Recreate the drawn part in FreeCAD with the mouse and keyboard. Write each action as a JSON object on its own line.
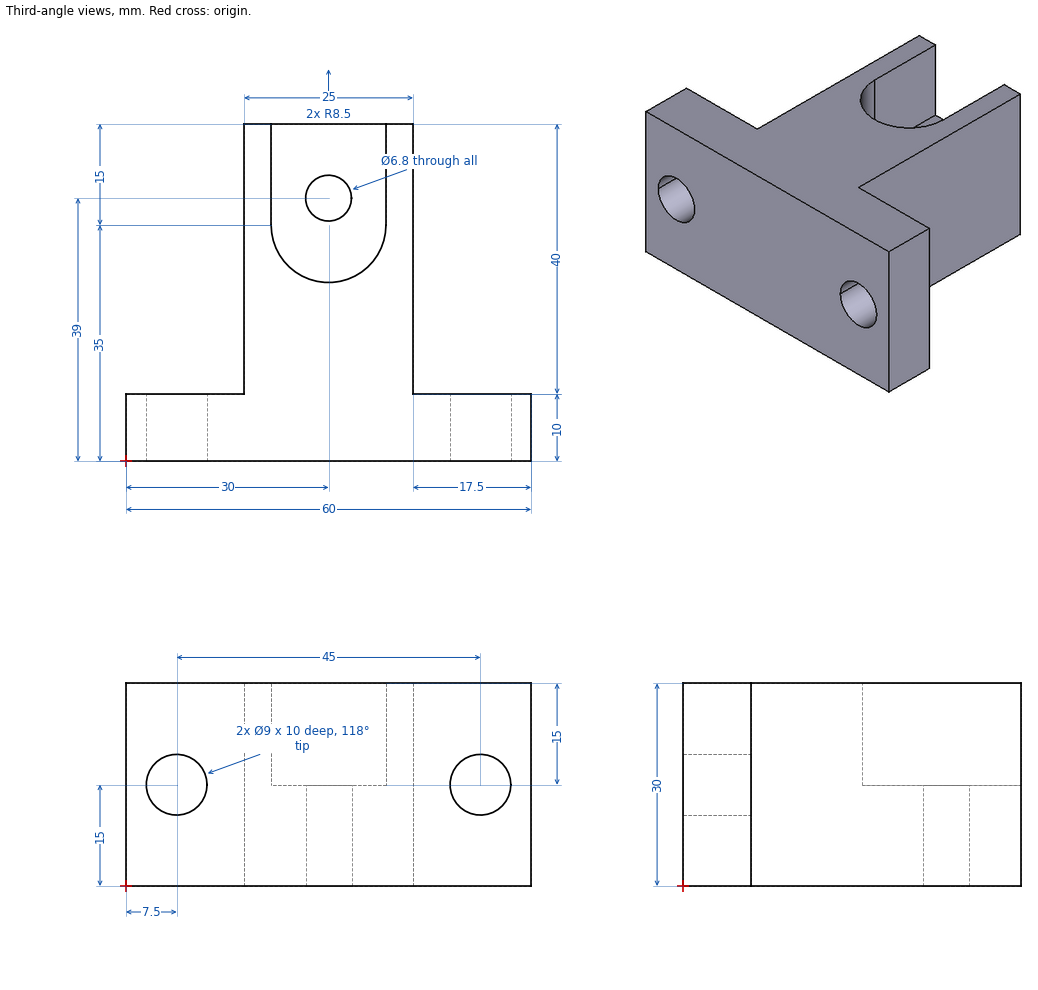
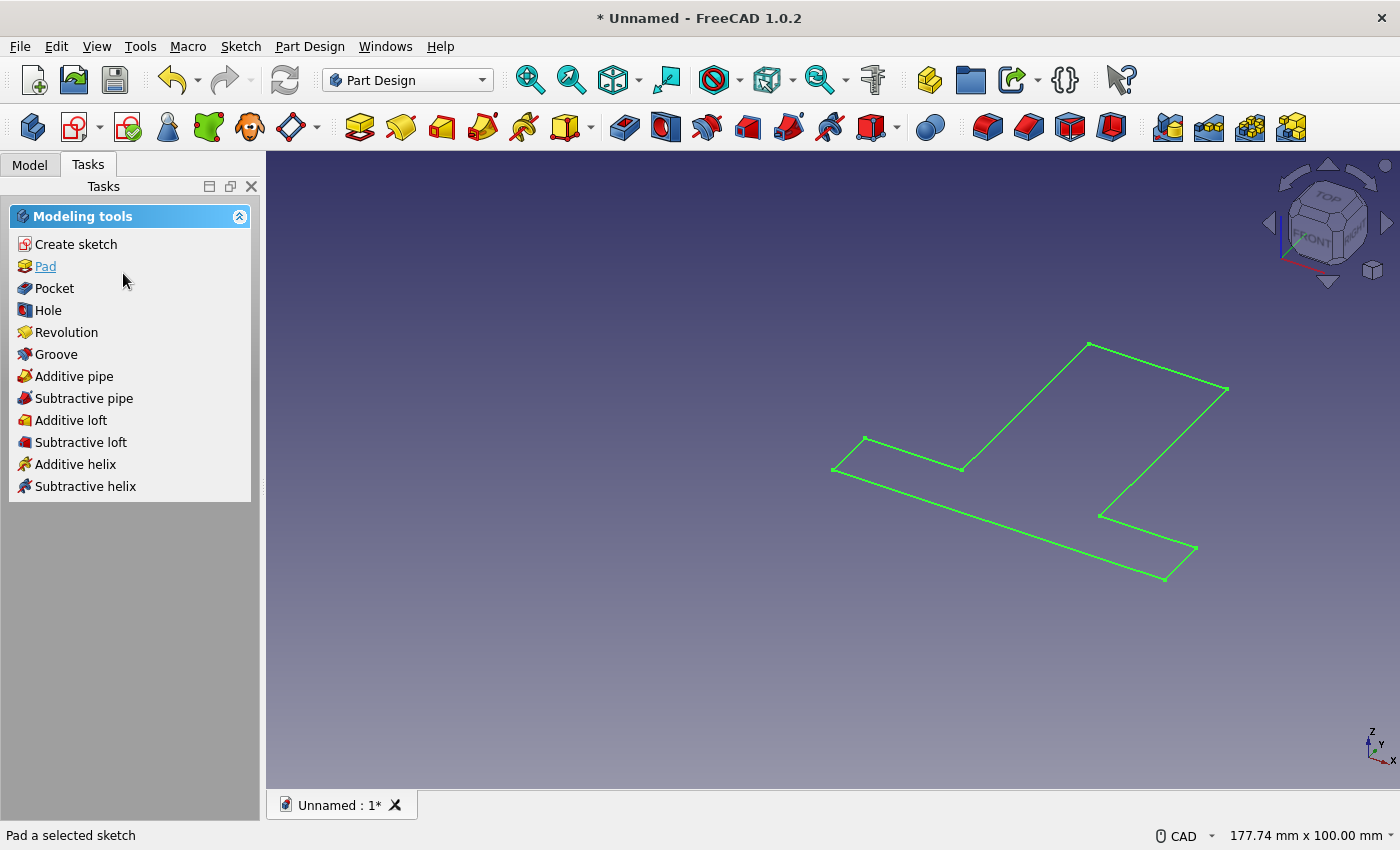
{"action": "left_click", "coordinate": [360, 128]}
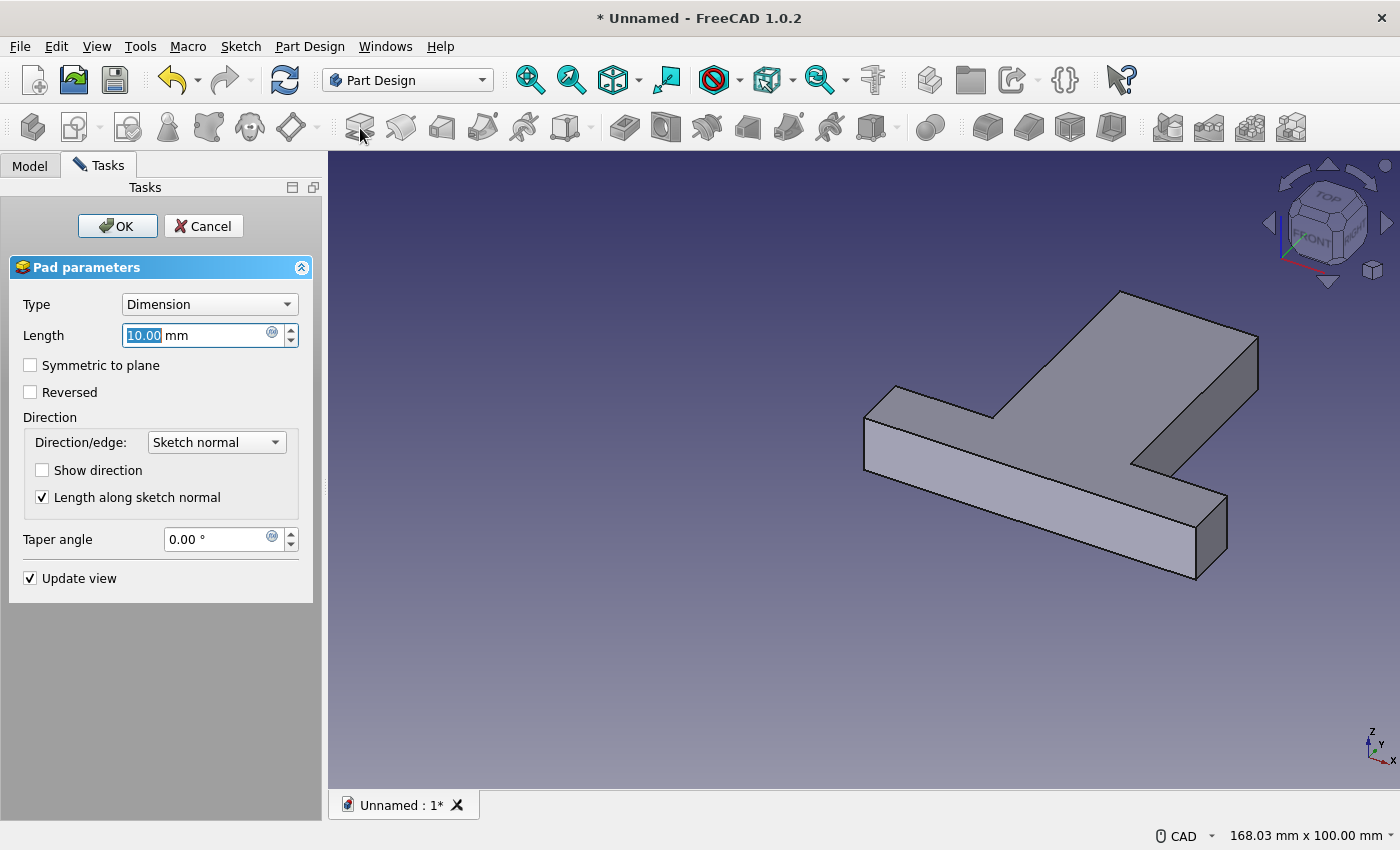
{"action": "type", "text": "30"}
{"action": "key", "text": "Tab"}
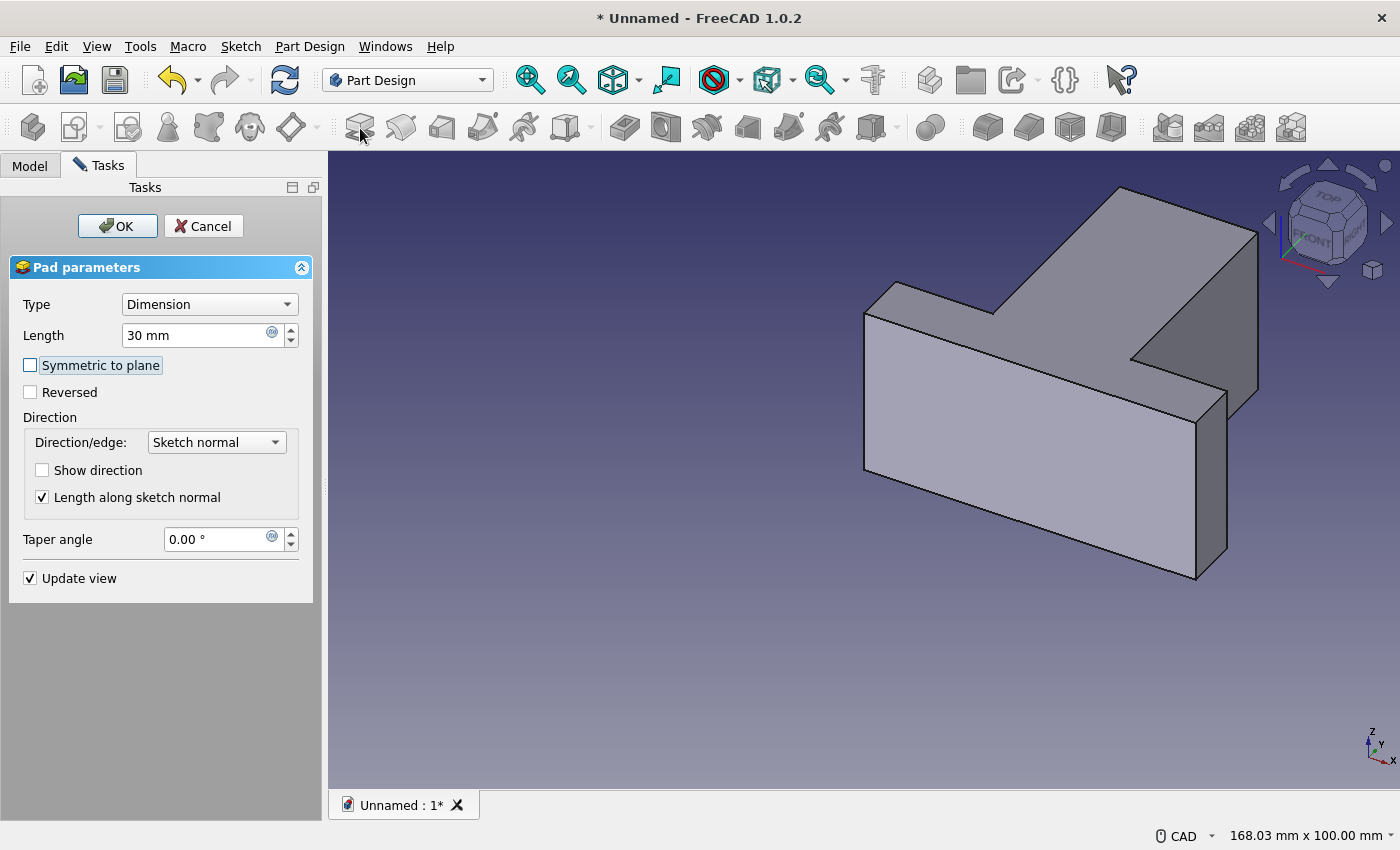
{"action": "left_click", "coordinate": [118, 226]}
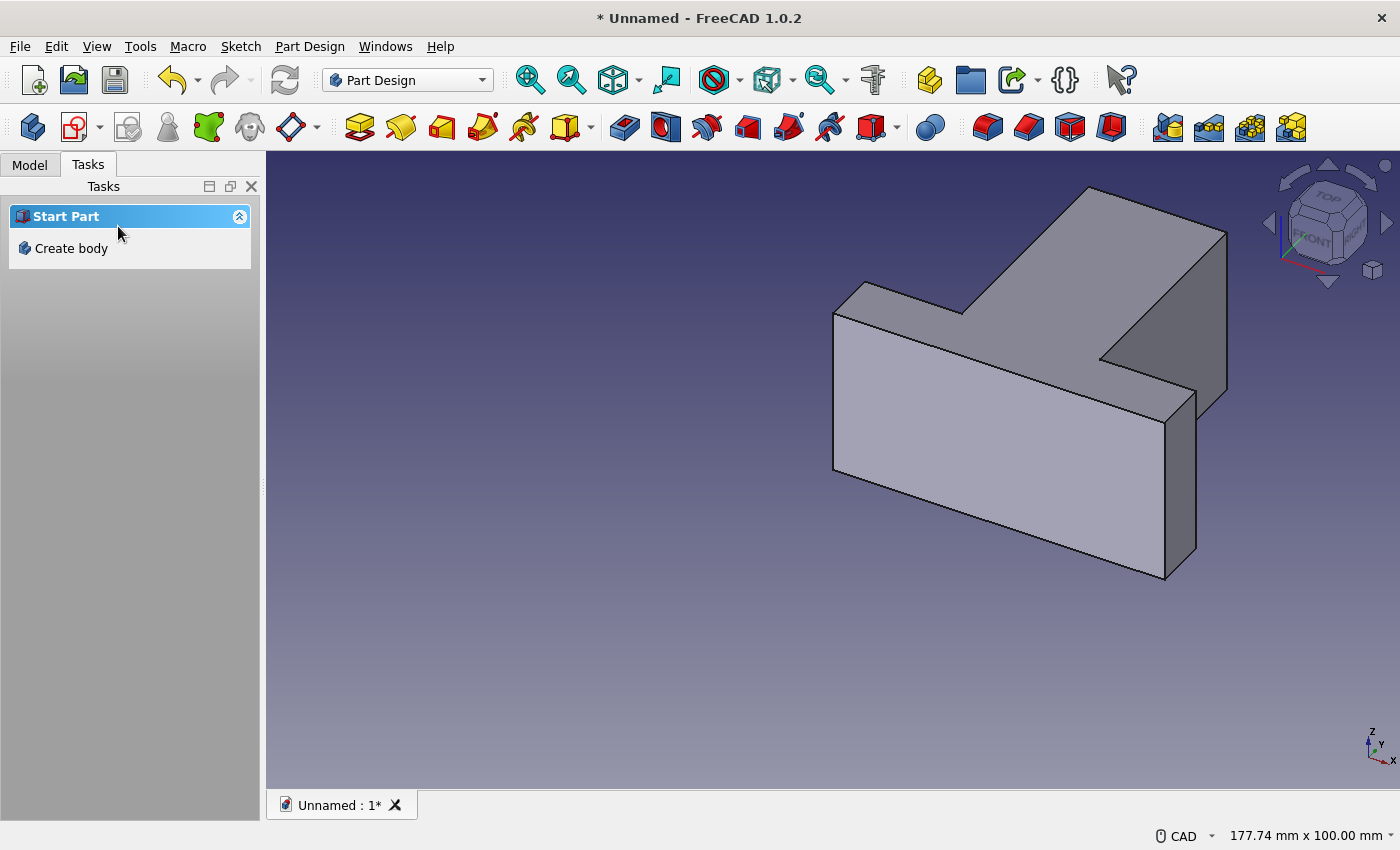
{"action": "left_click", "coordinate": [1101, 265]}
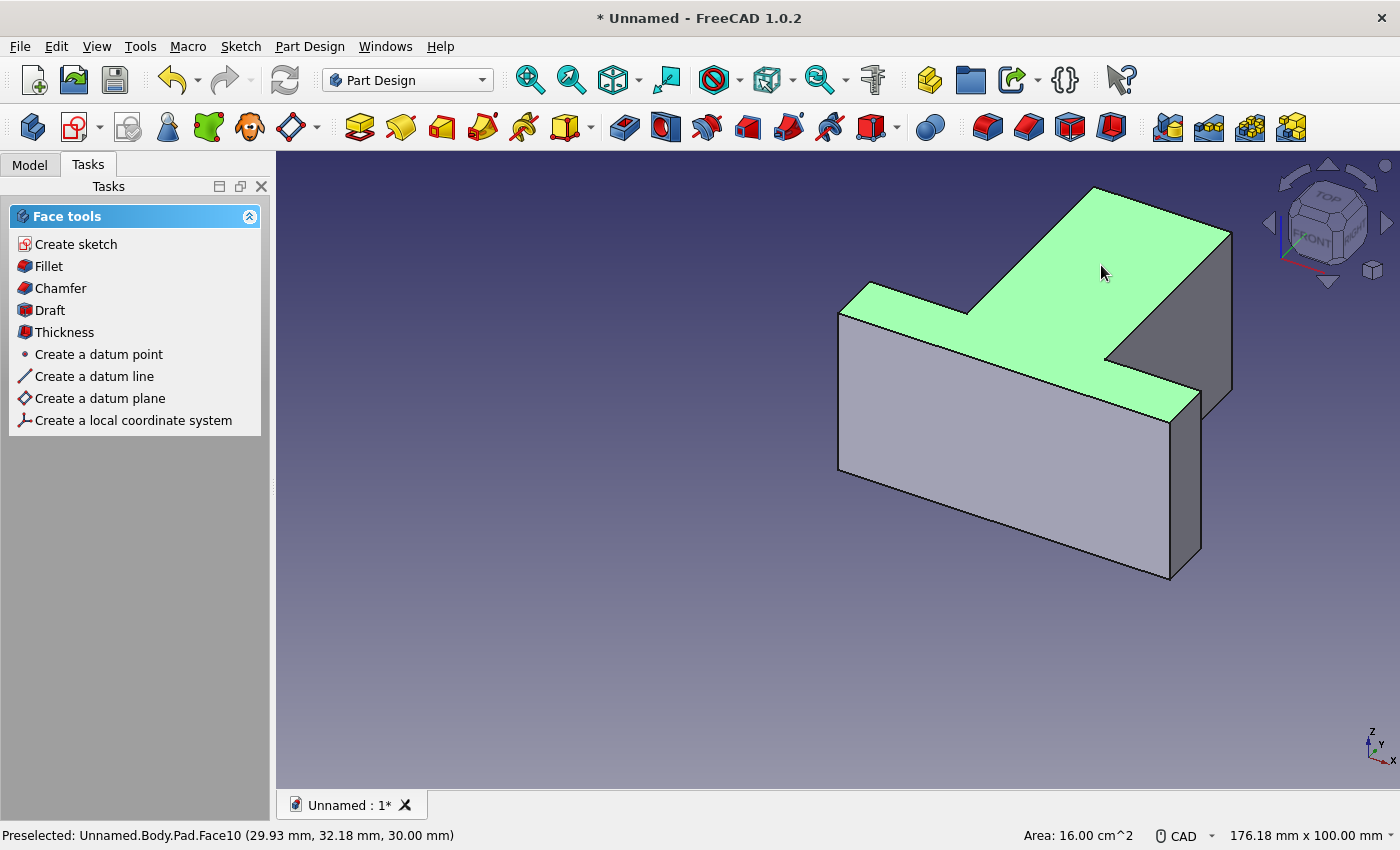
{"action": "left_click", "coordinate": [74, 128]}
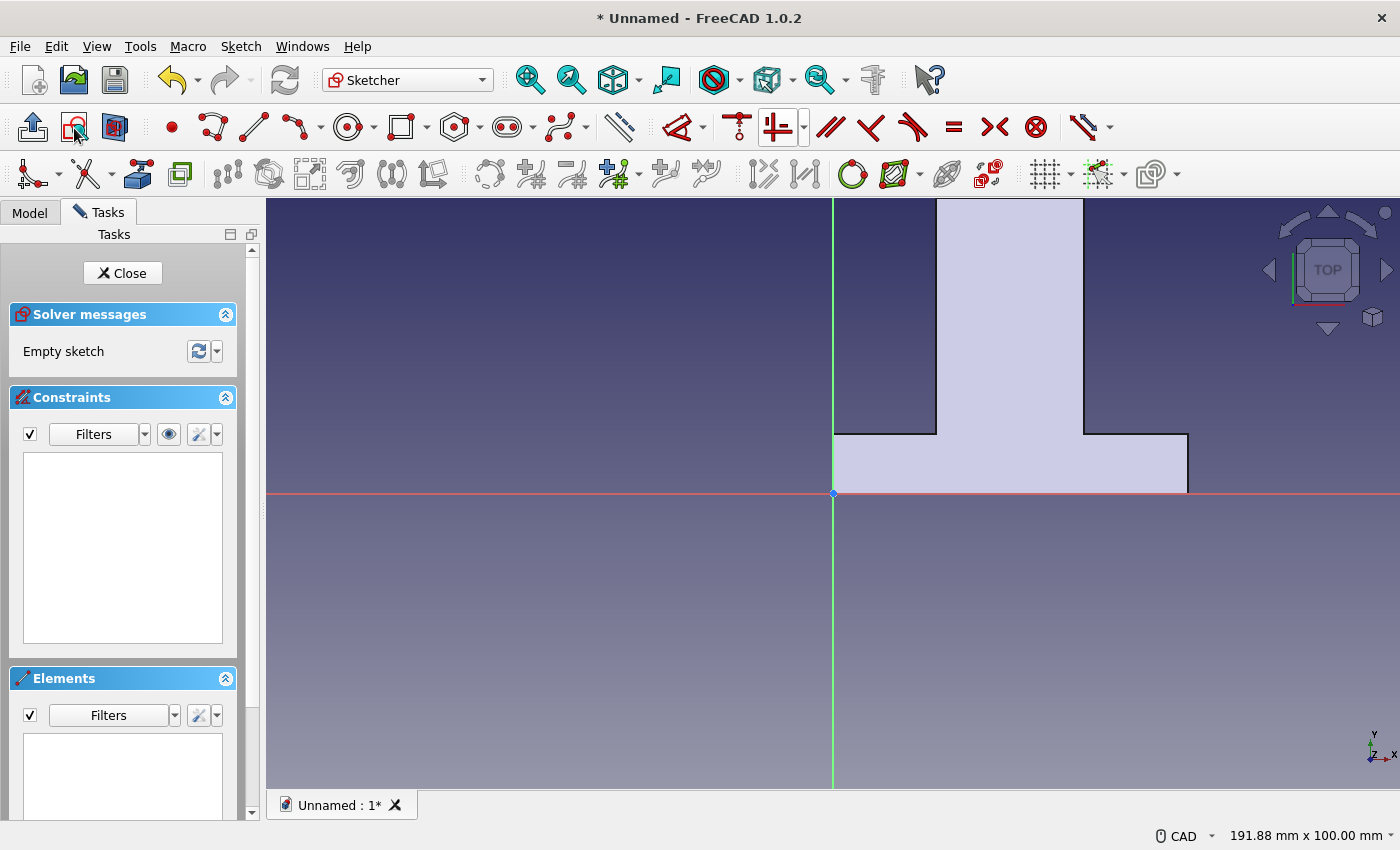
{"action": "scroll", "coordinate": [294, 761], "scroll_direction": "down", "scroll_amount": 1}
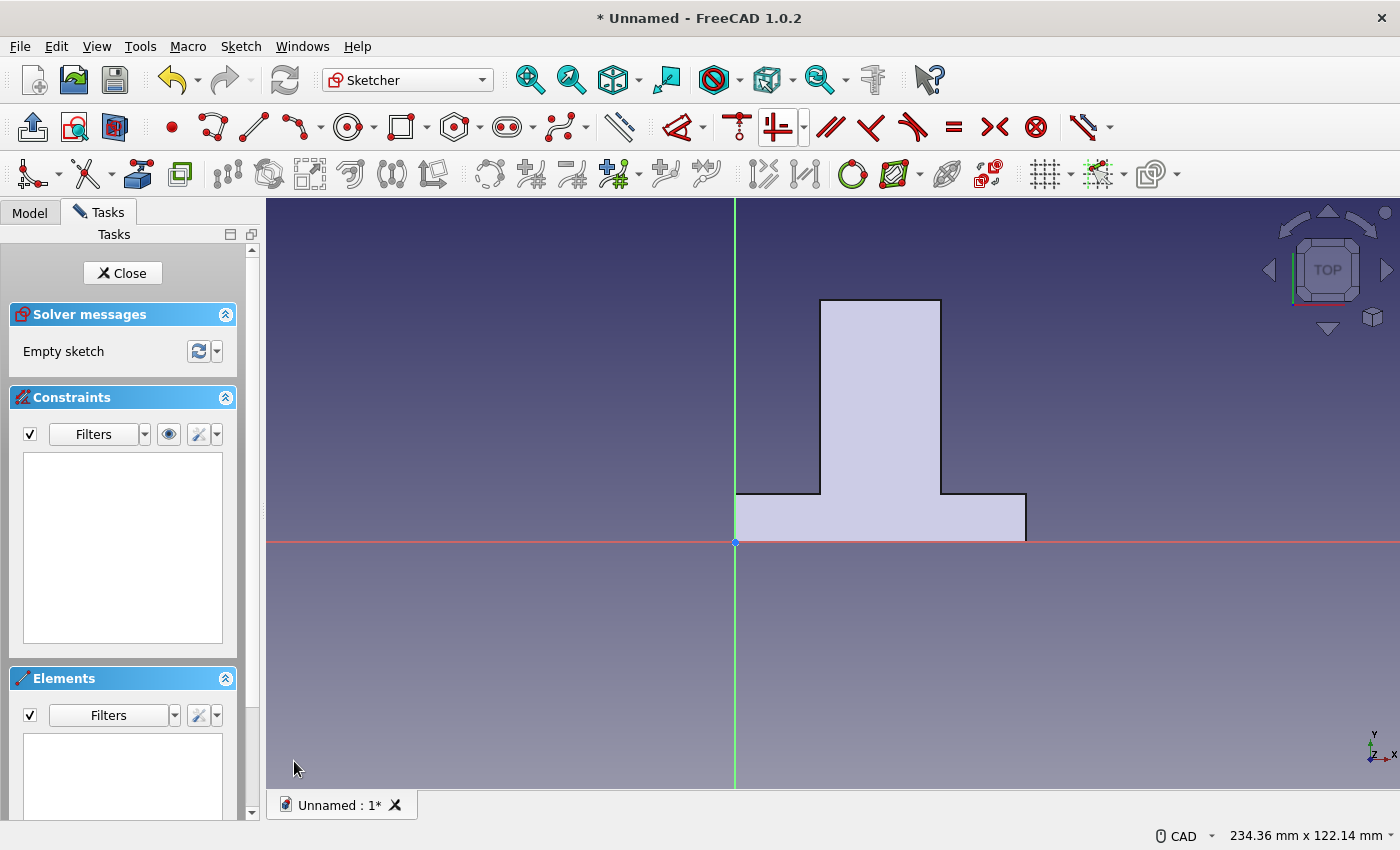
{"action": "key", "text": "g s"}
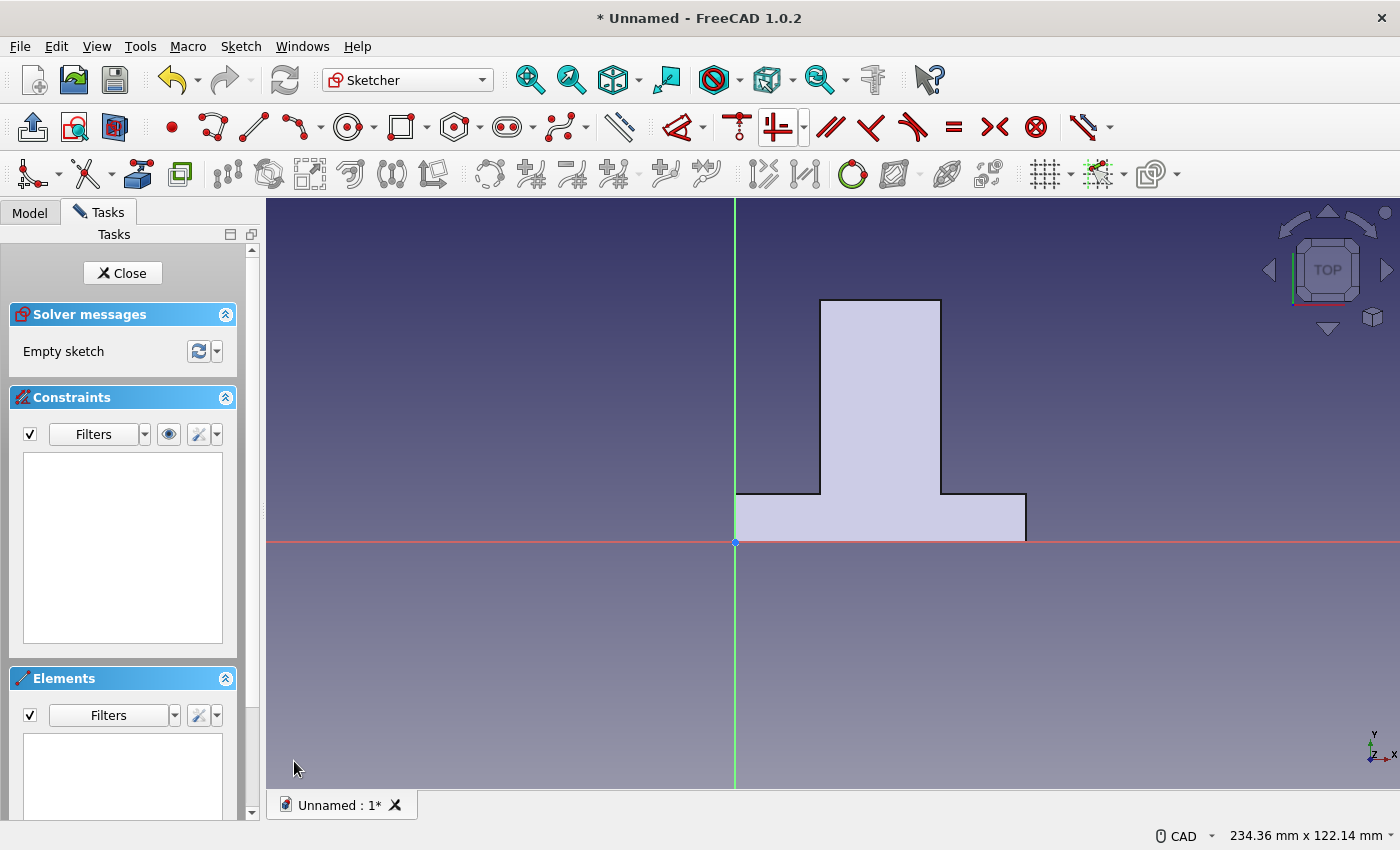
{"action": "left_click", "coordinate": [880, 373]}